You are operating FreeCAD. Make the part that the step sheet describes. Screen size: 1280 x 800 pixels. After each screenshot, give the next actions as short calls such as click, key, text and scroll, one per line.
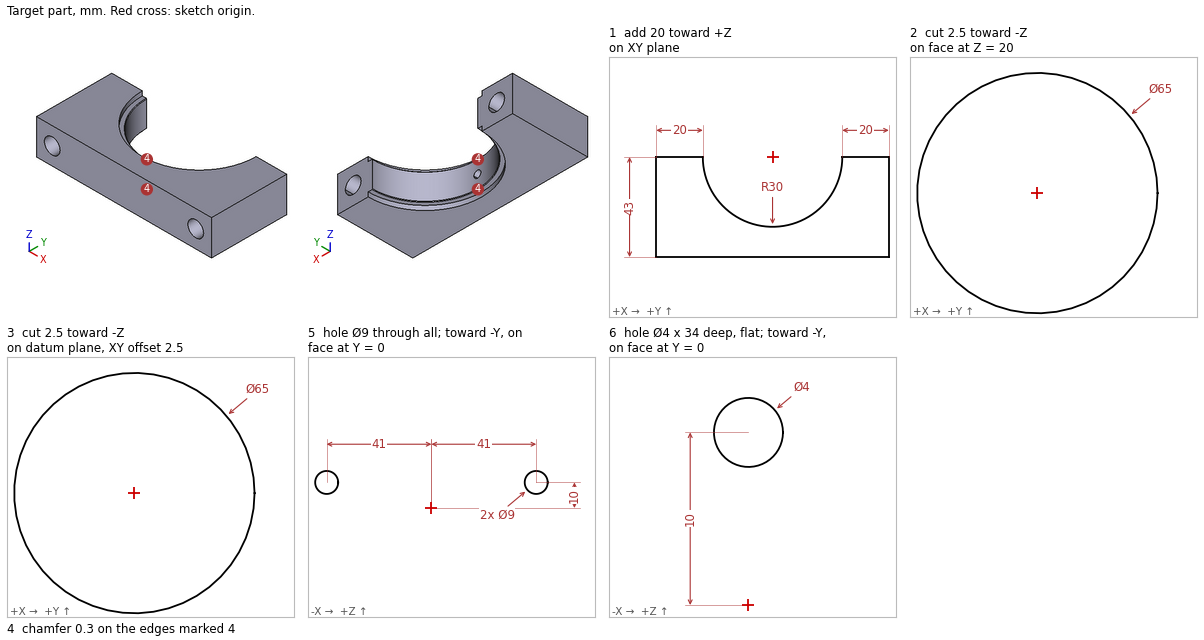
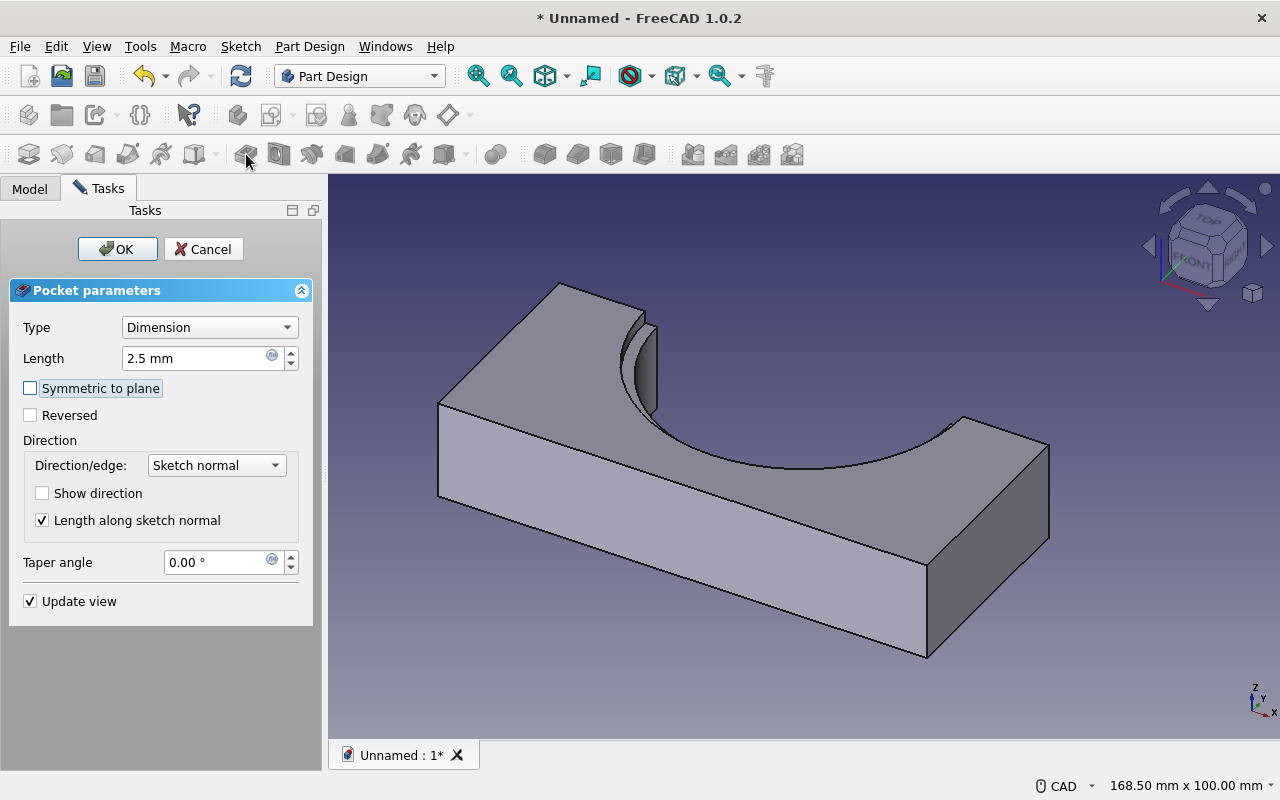
click(118, 249)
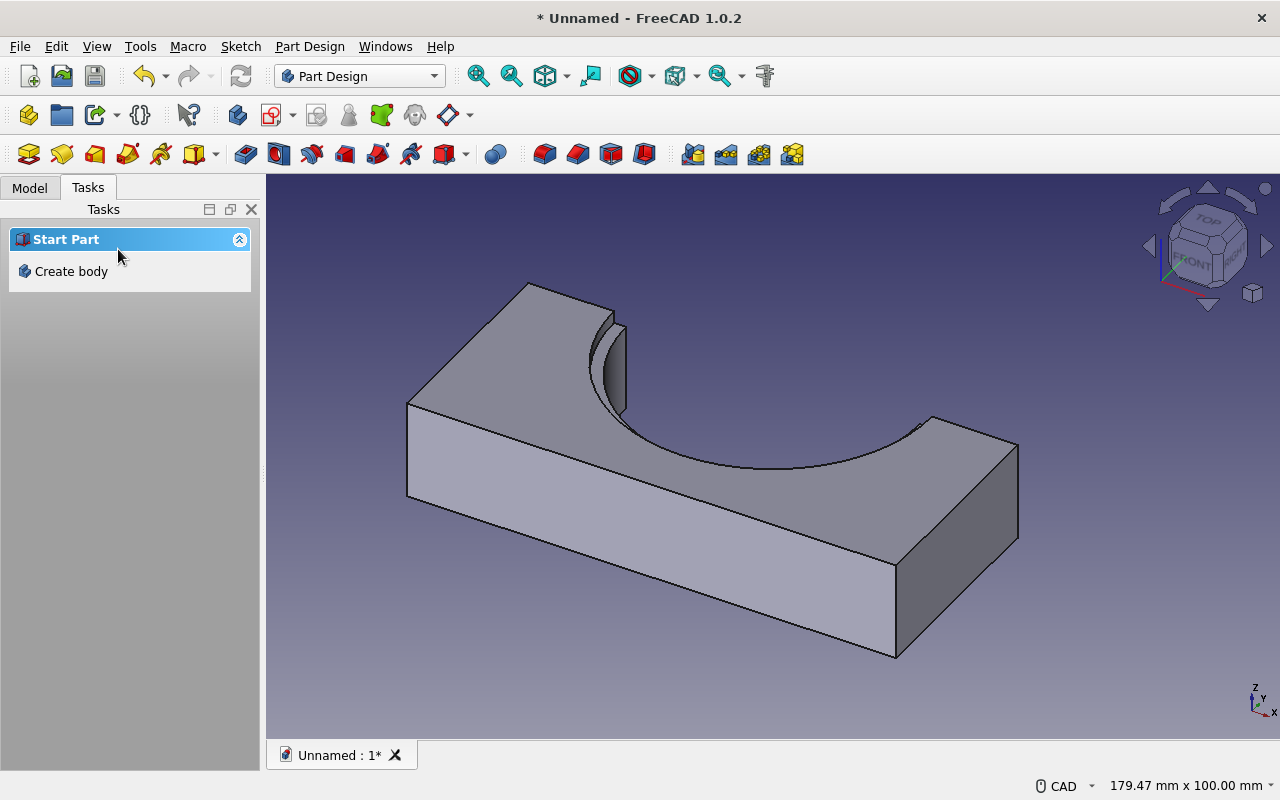
click(30, 188)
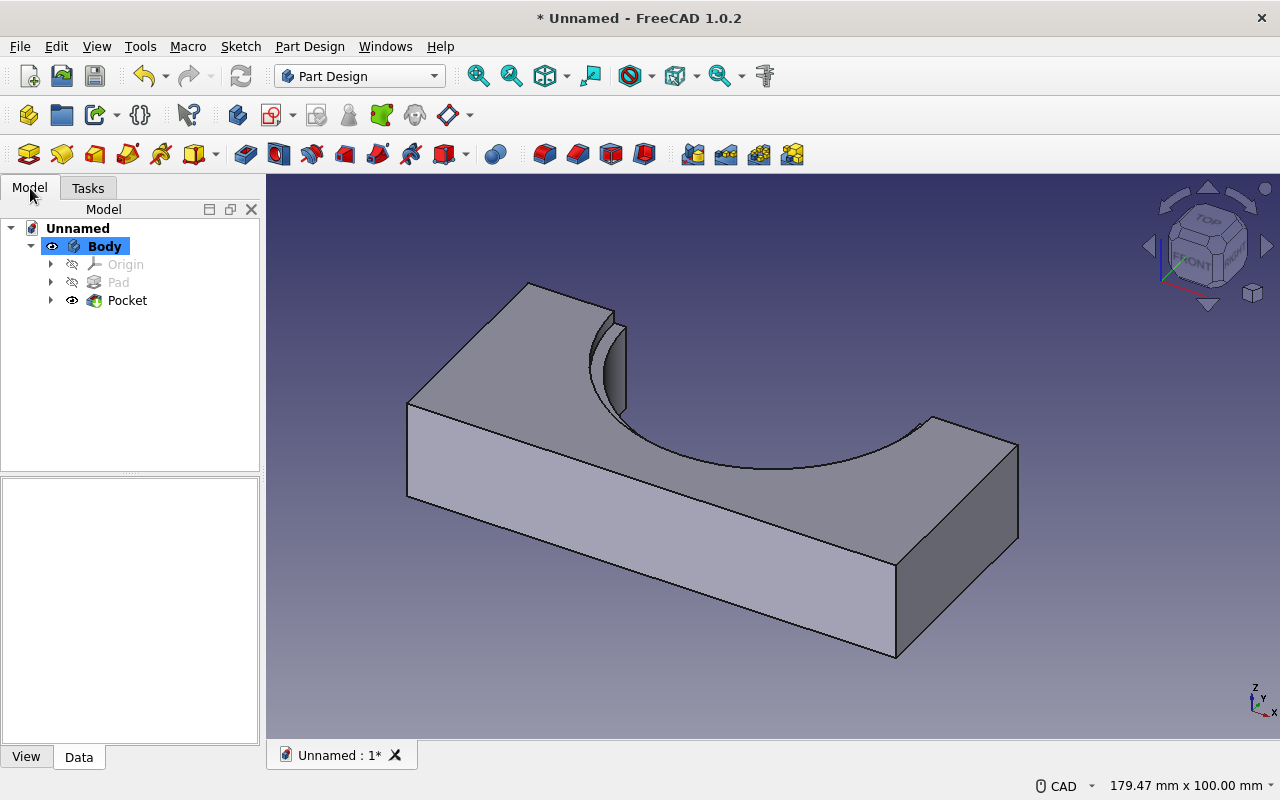
click(51, 264)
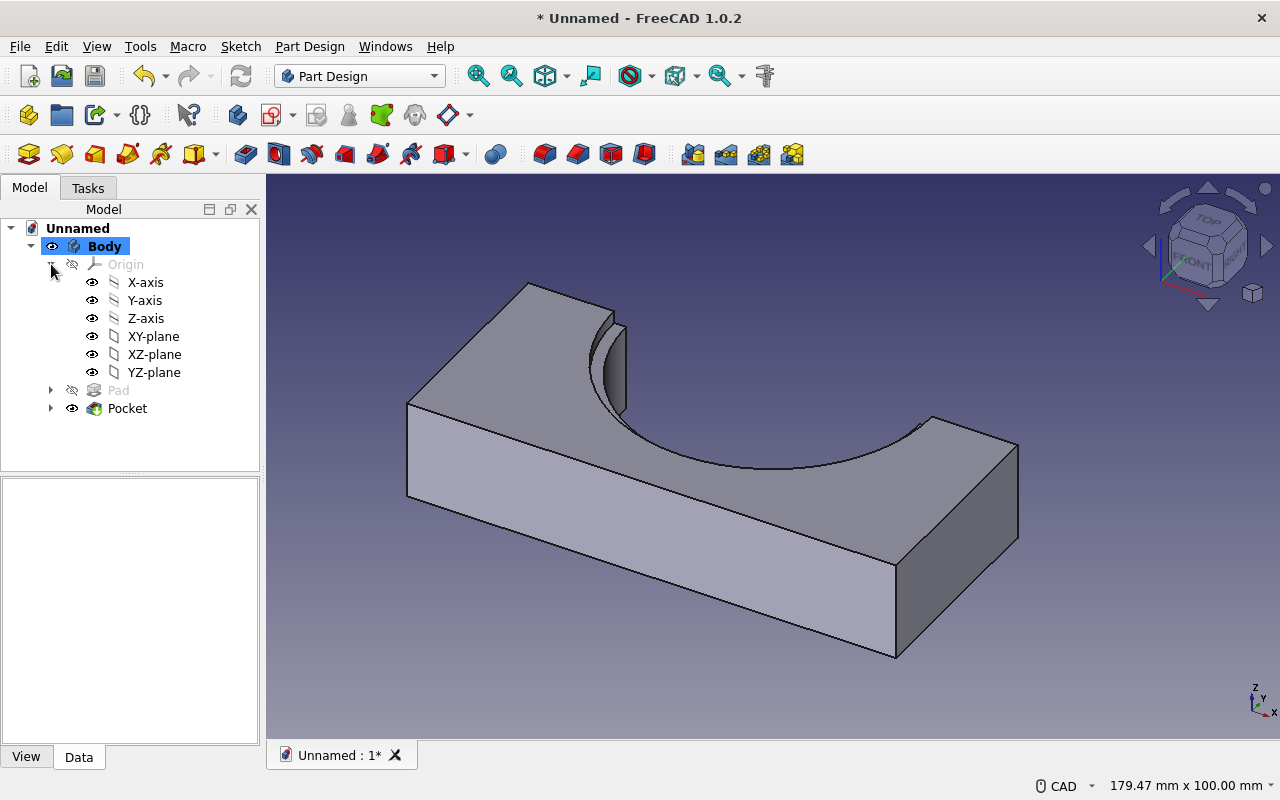
click(137, 336)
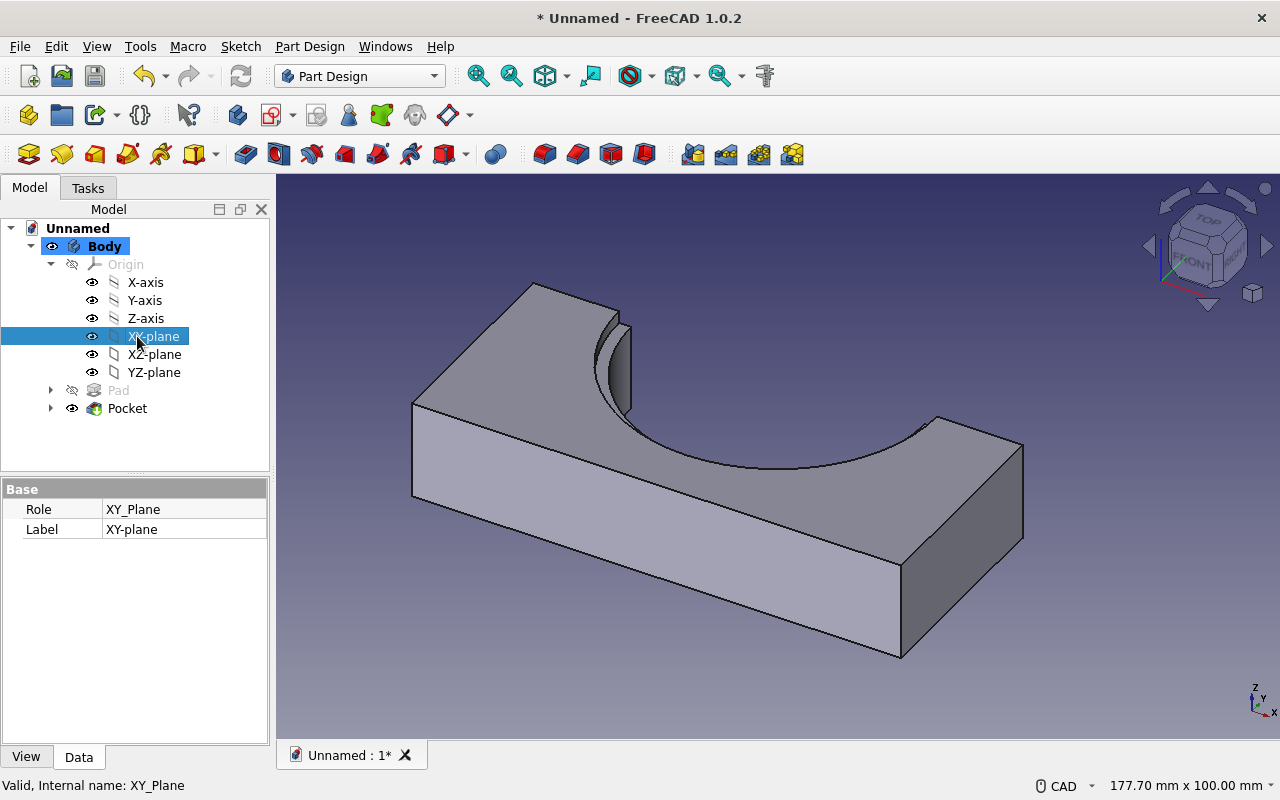
click(448, 116)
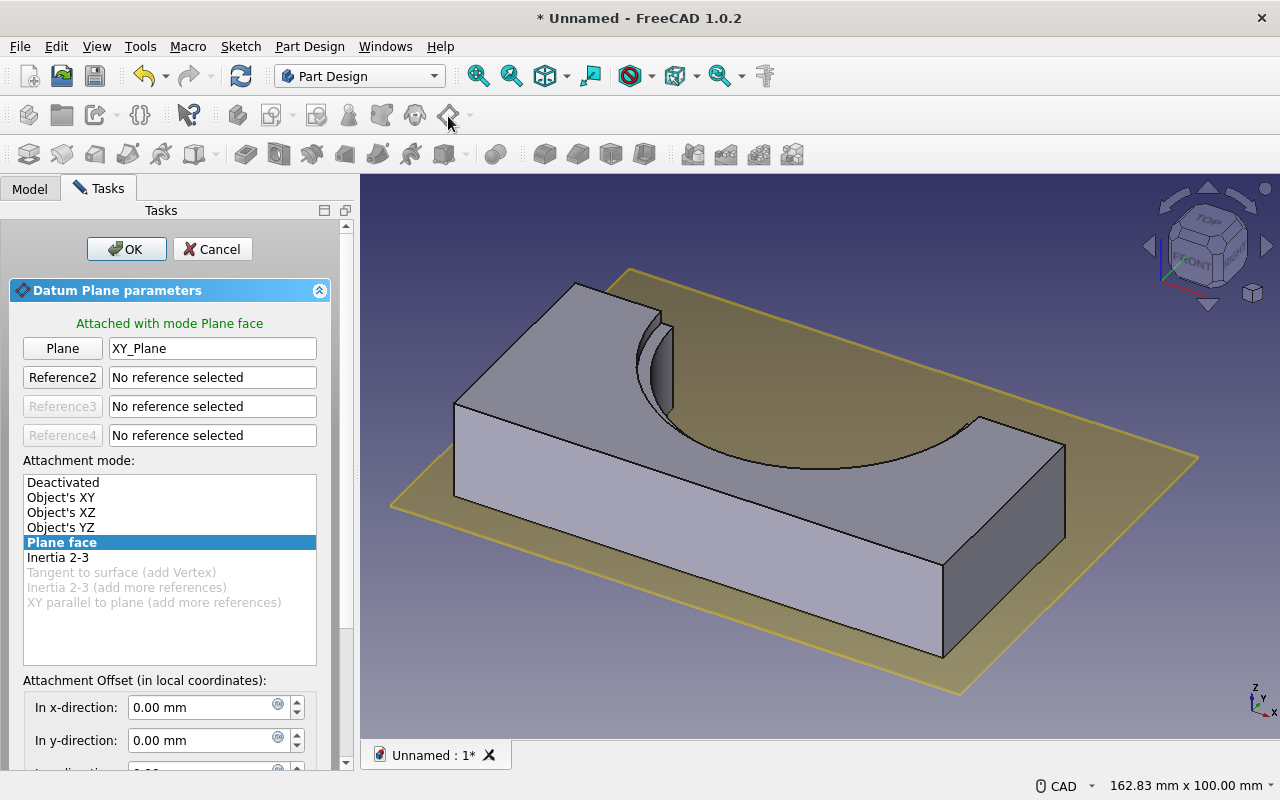
scroll(346, 495, down, 2)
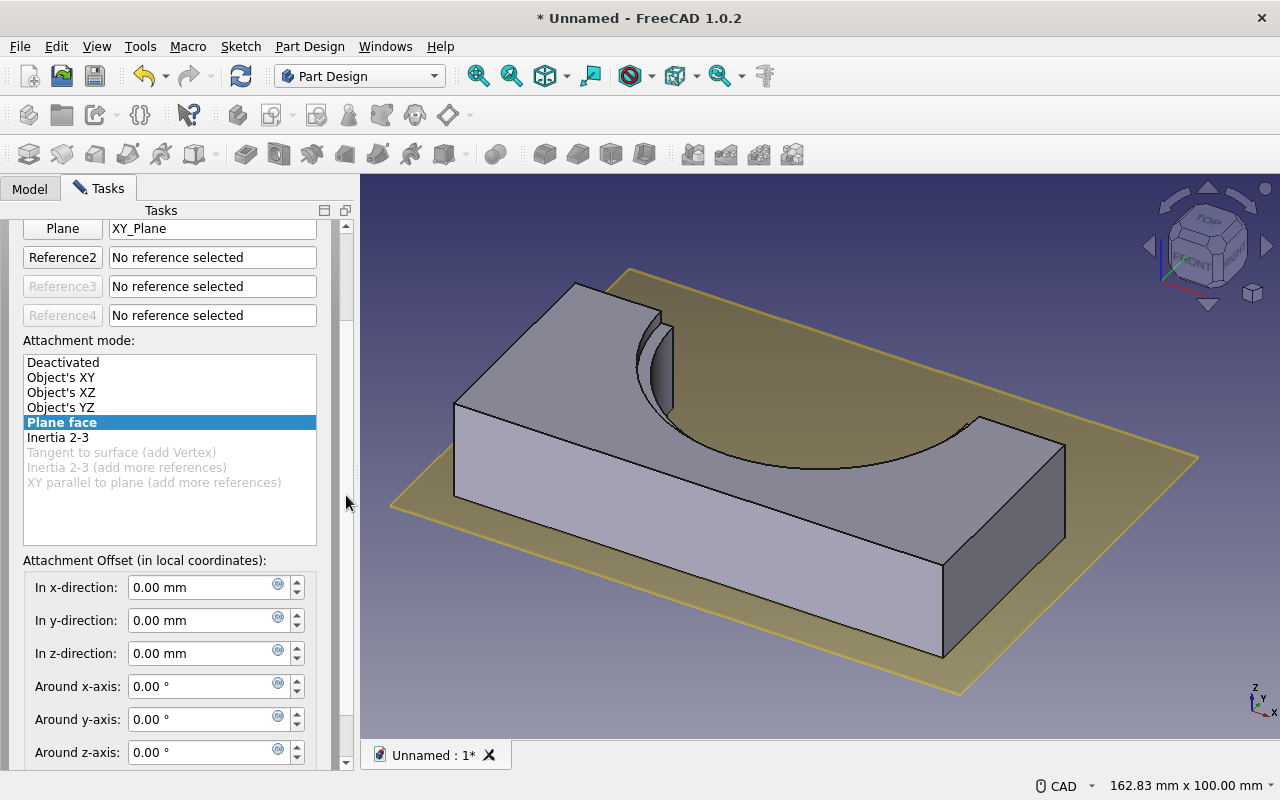
triple_click(210, 654)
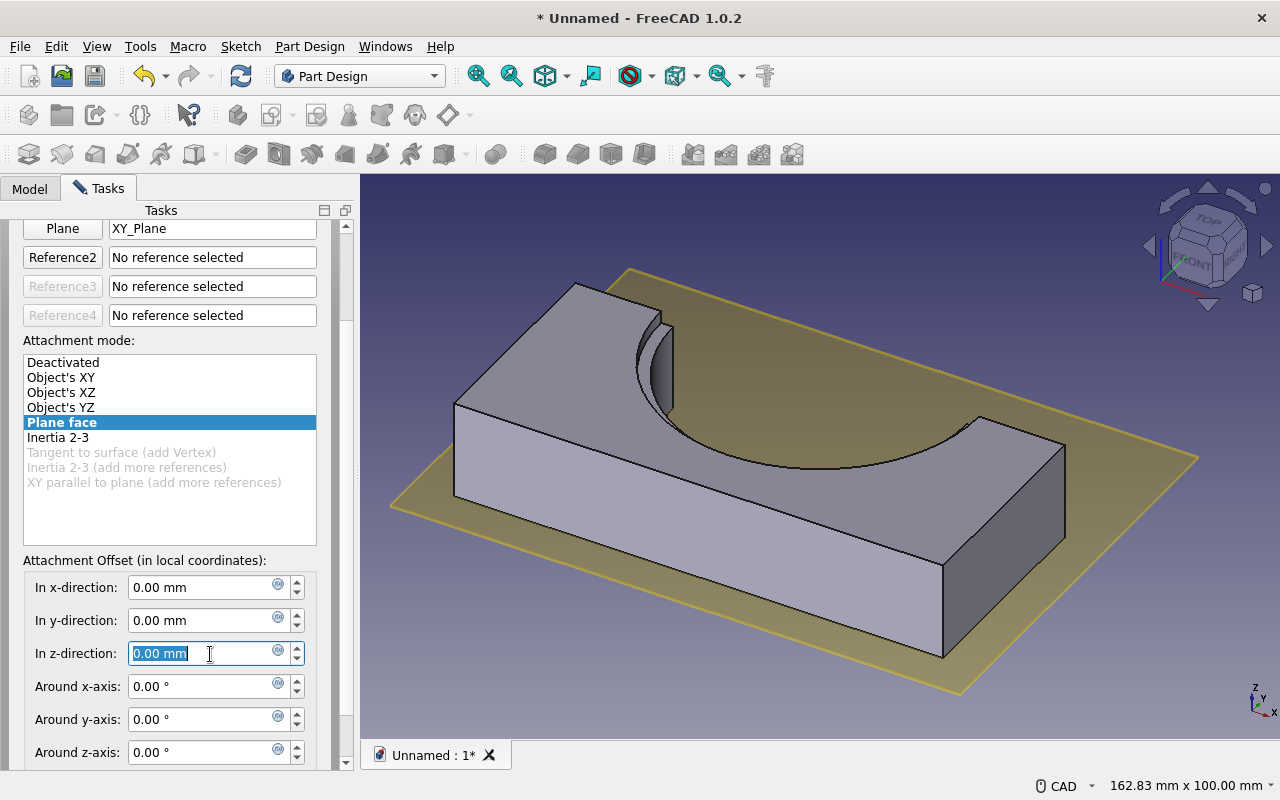
text(2.5)
key(Tab)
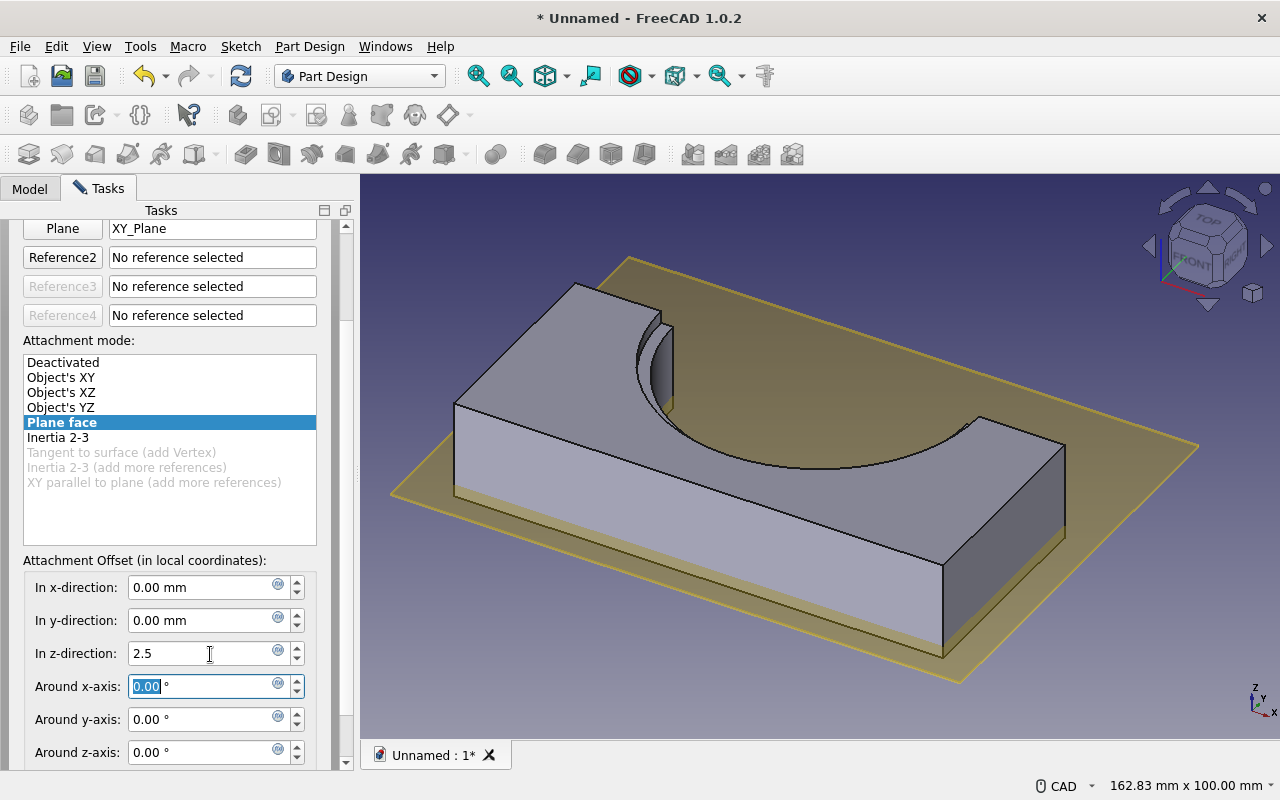
scroll(346, 495, up, 3)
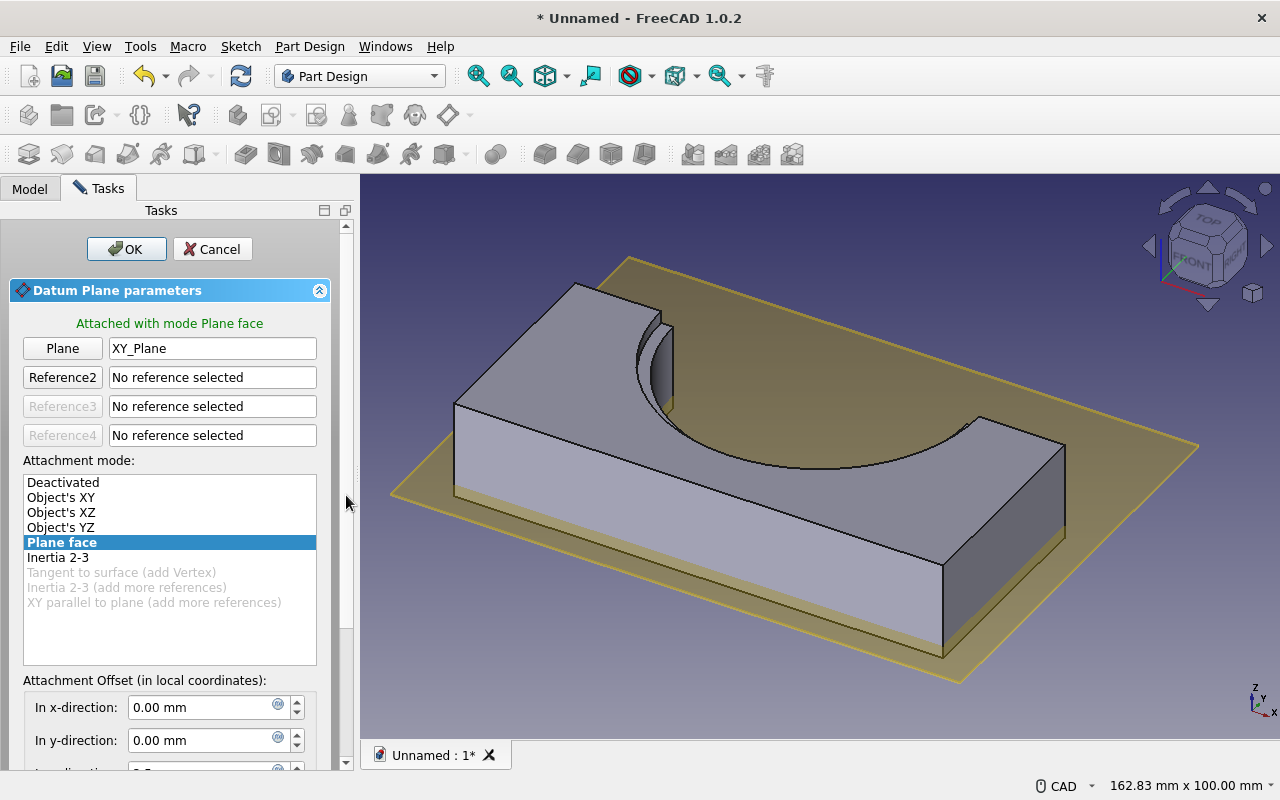
click(127, 249)